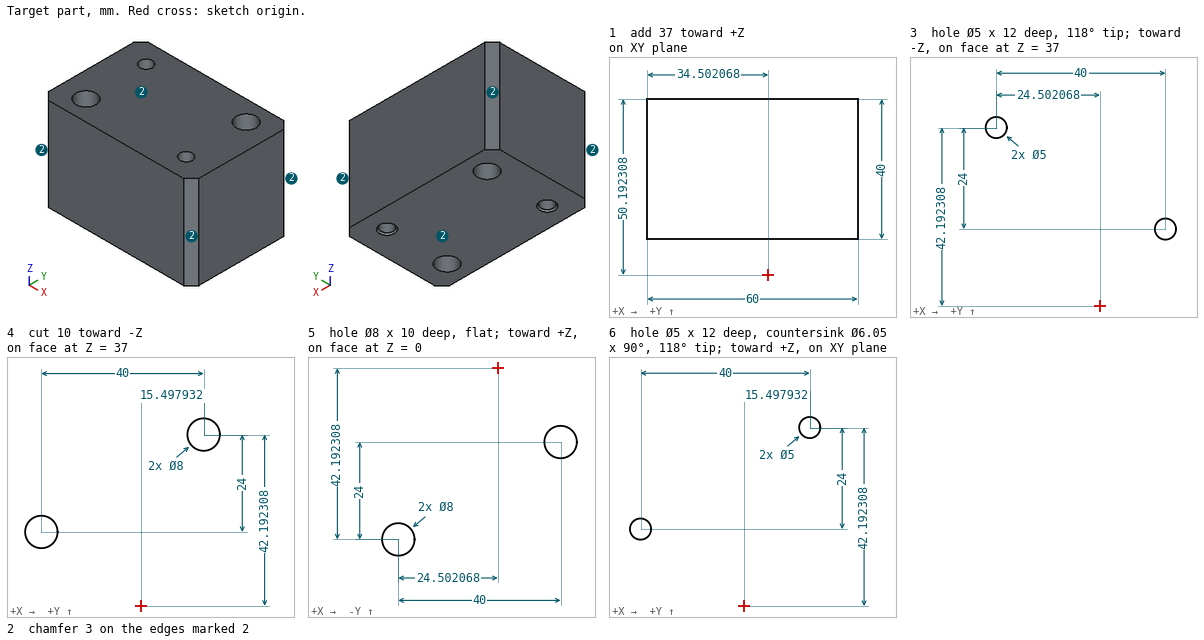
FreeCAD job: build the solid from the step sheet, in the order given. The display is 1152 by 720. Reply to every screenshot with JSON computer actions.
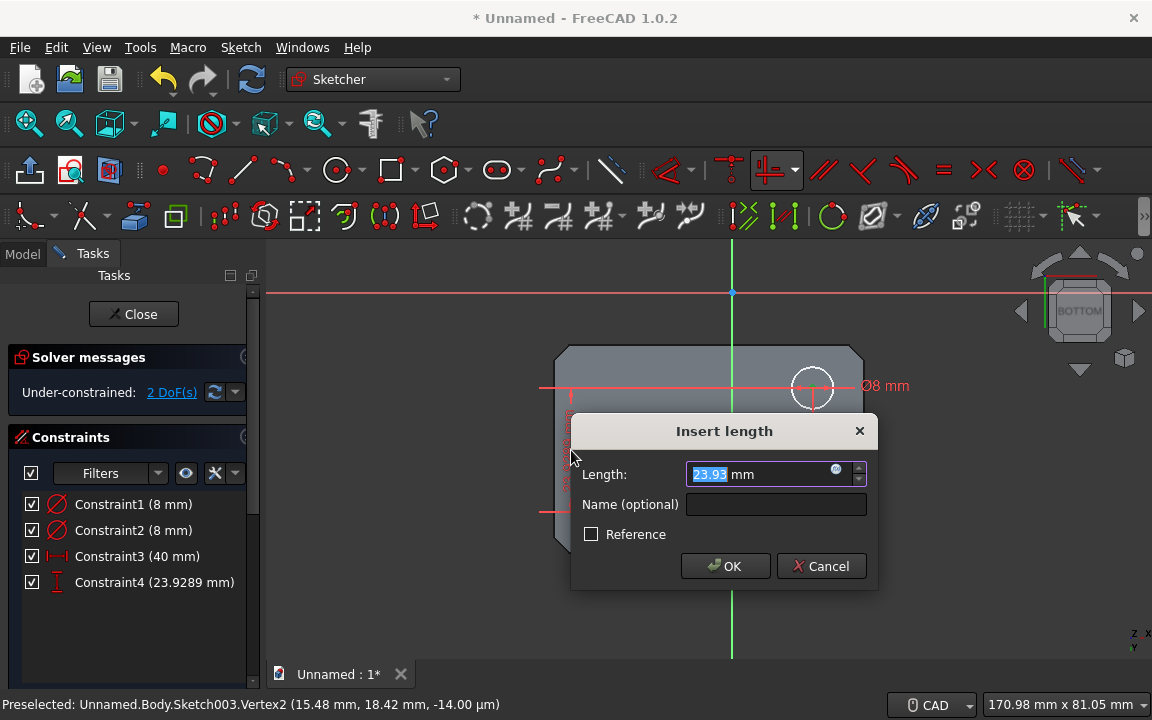
{"action": "type", "text": "24"}
{"action": "key", "text": "Return"}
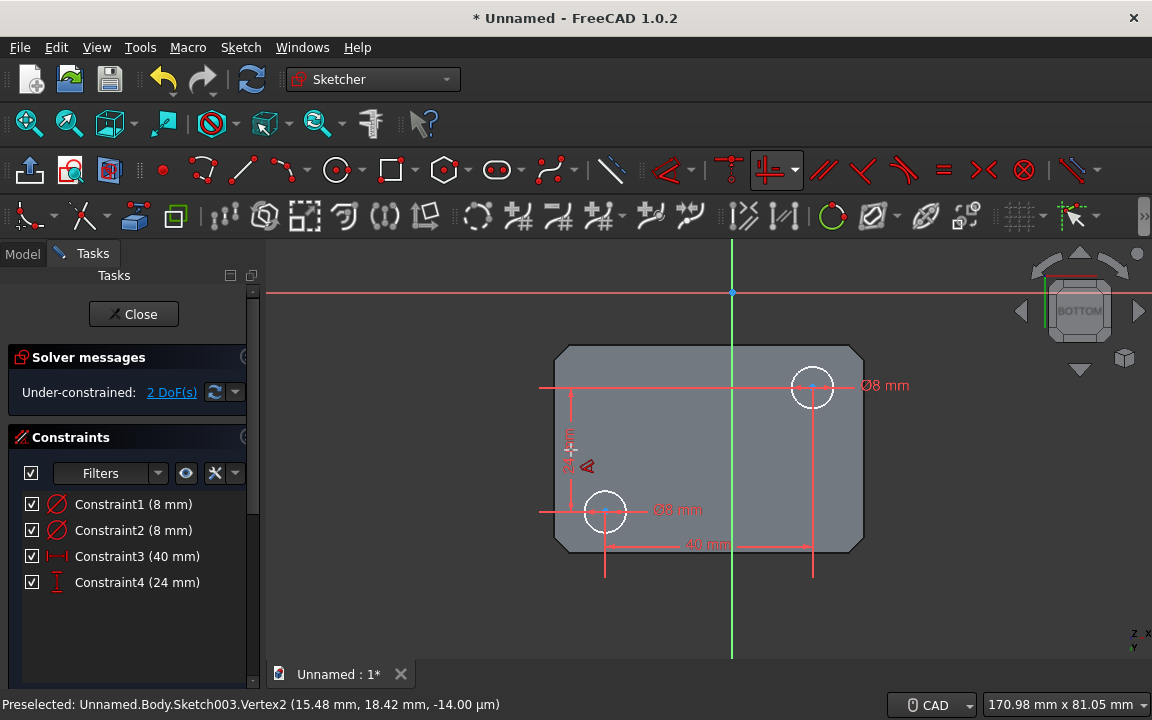
{"action": "left_click", "coordinate": [605, 512]}
{"action": "left_click", "coordinate": [624, 546]}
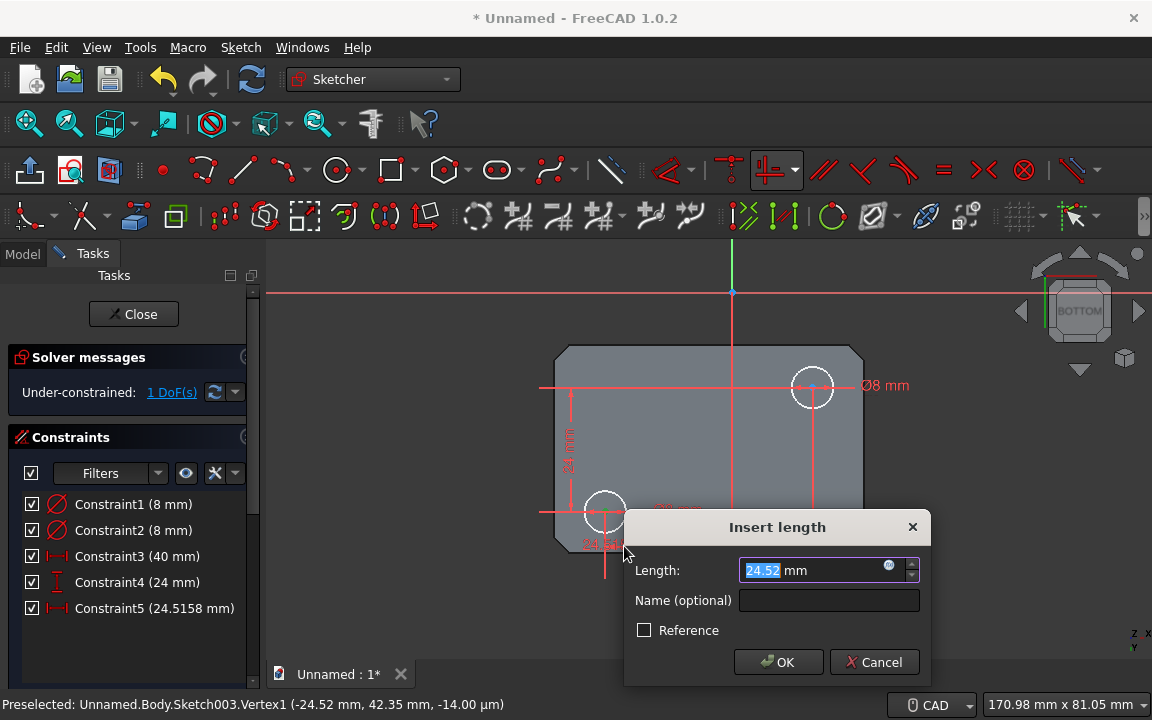
{"action": "type", "text": "24.502068"}
{"action": "key", "text": "Return"}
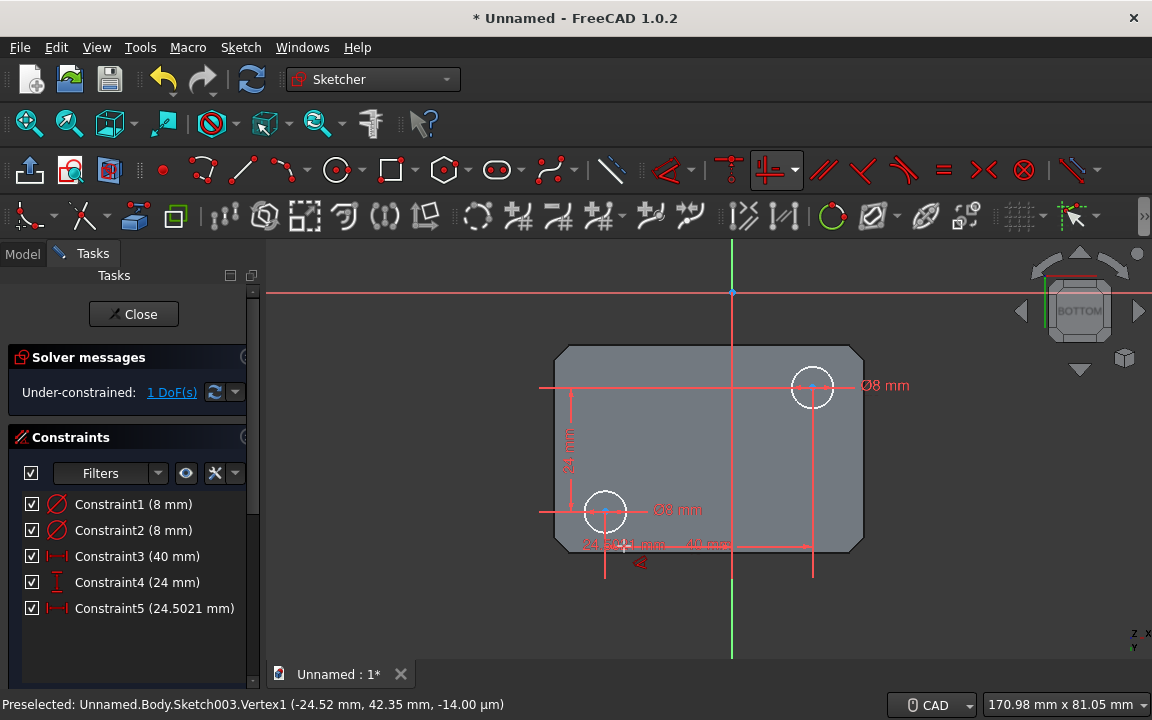
{"action": "left_click", "coordinate": [605, 512]}
{"action": "left_click", "coordinate": [571, 402]}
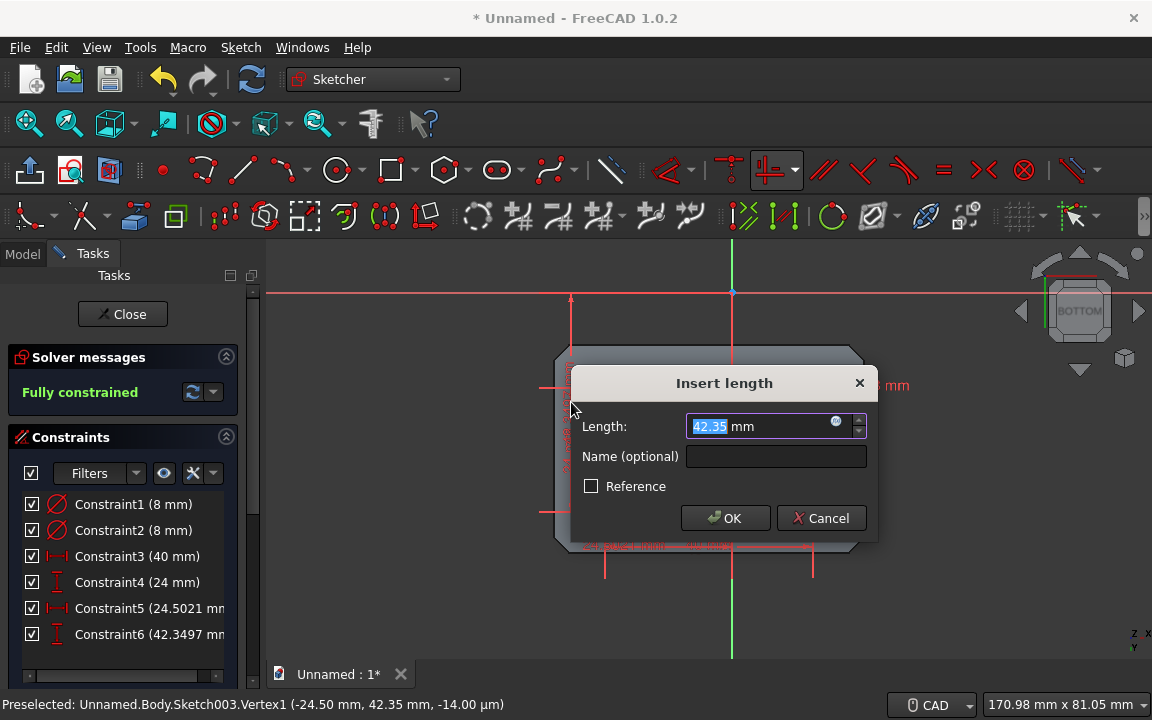
{"action": "type", "text": "42.192308"}
{"action": "key", "text": "Return"}
{"action": "key", "text": "Escape"}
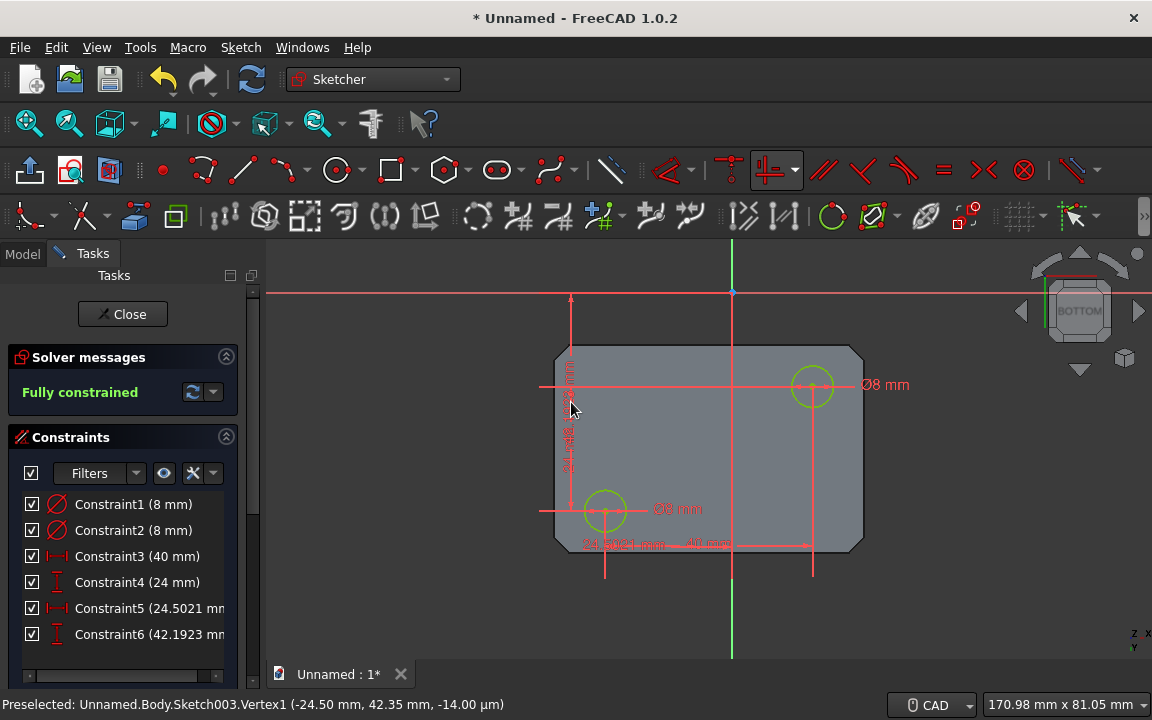
{"action": "left_click", "coordinate": [123, 314]}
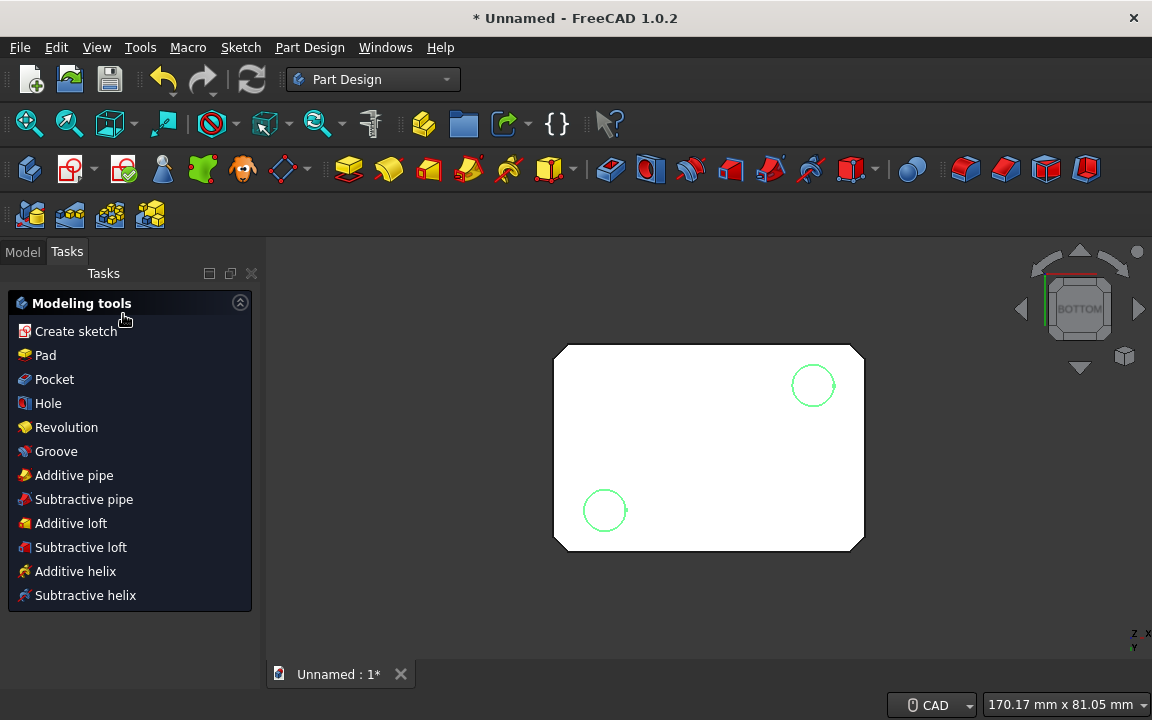
{"action": "left_click", "coordinate": [652, 170]}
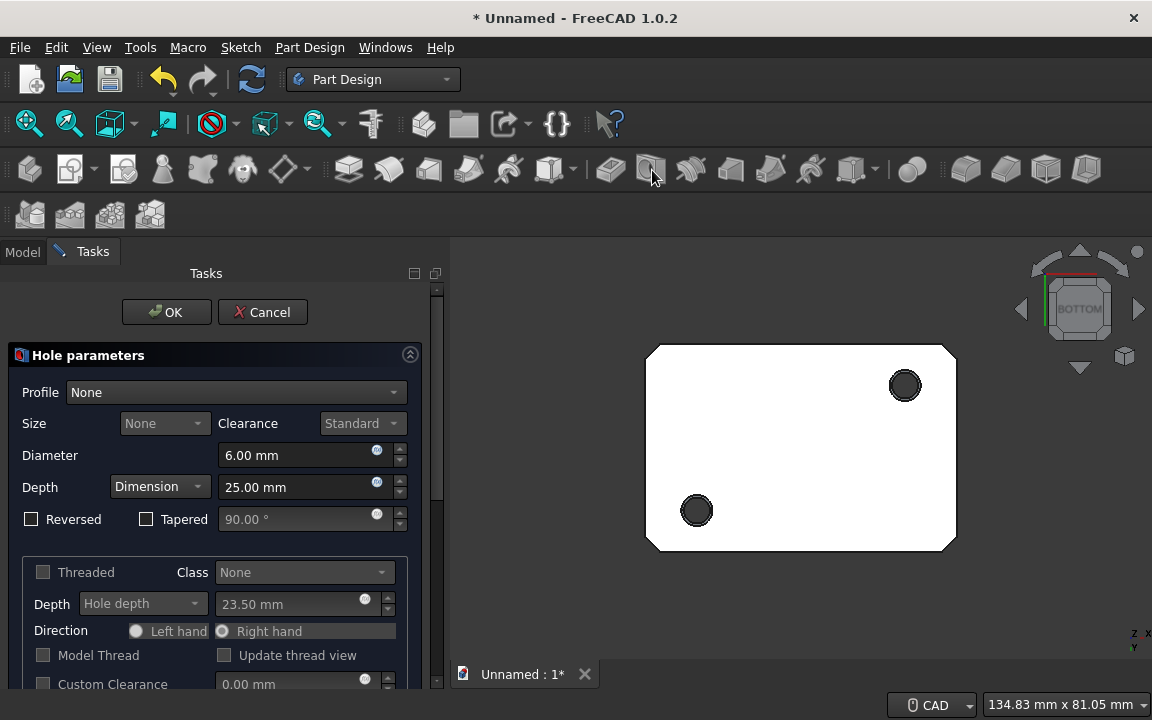
{"action": "triple_click", "coordinate": [305, 455]}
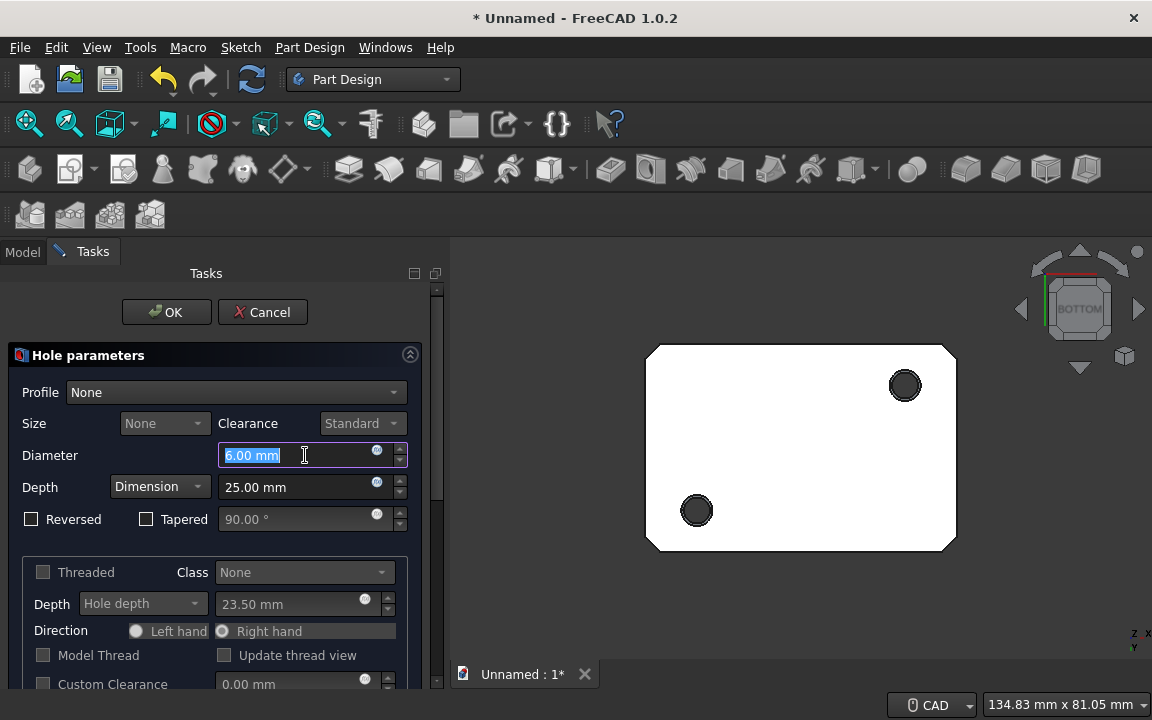
{"action": "type", "text": "8"}
{"action": "key", "text": "Tab"}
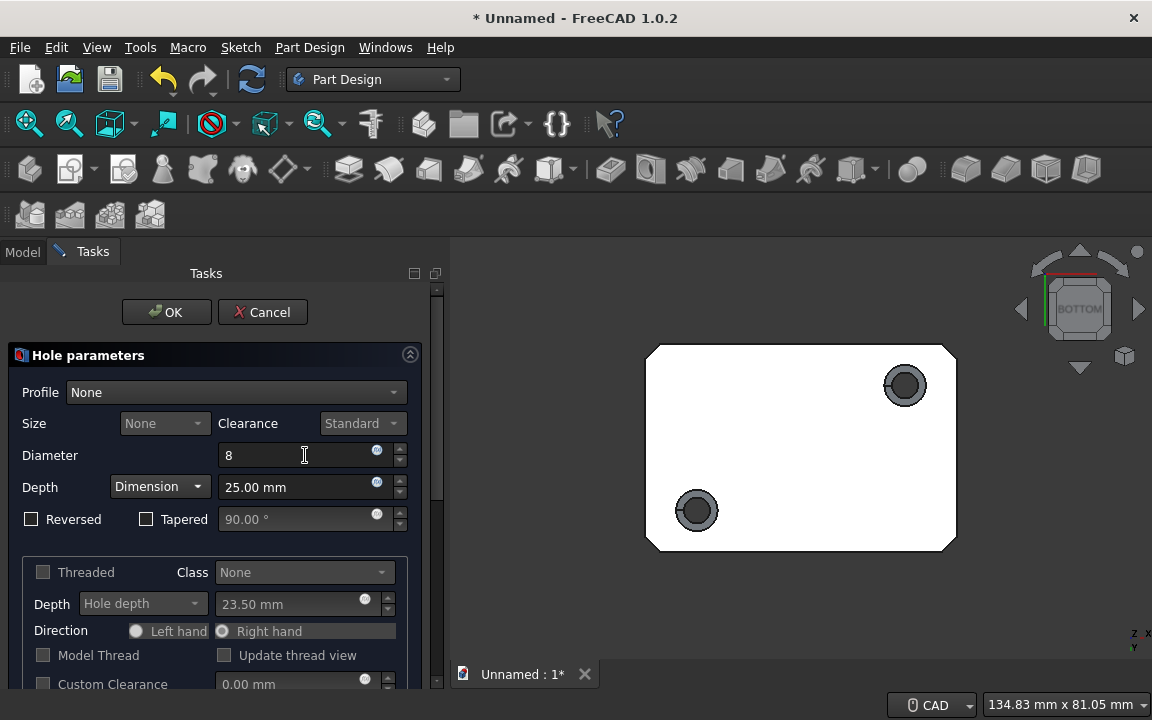
{"action": "triple_click", "coordinate": [305, 487]}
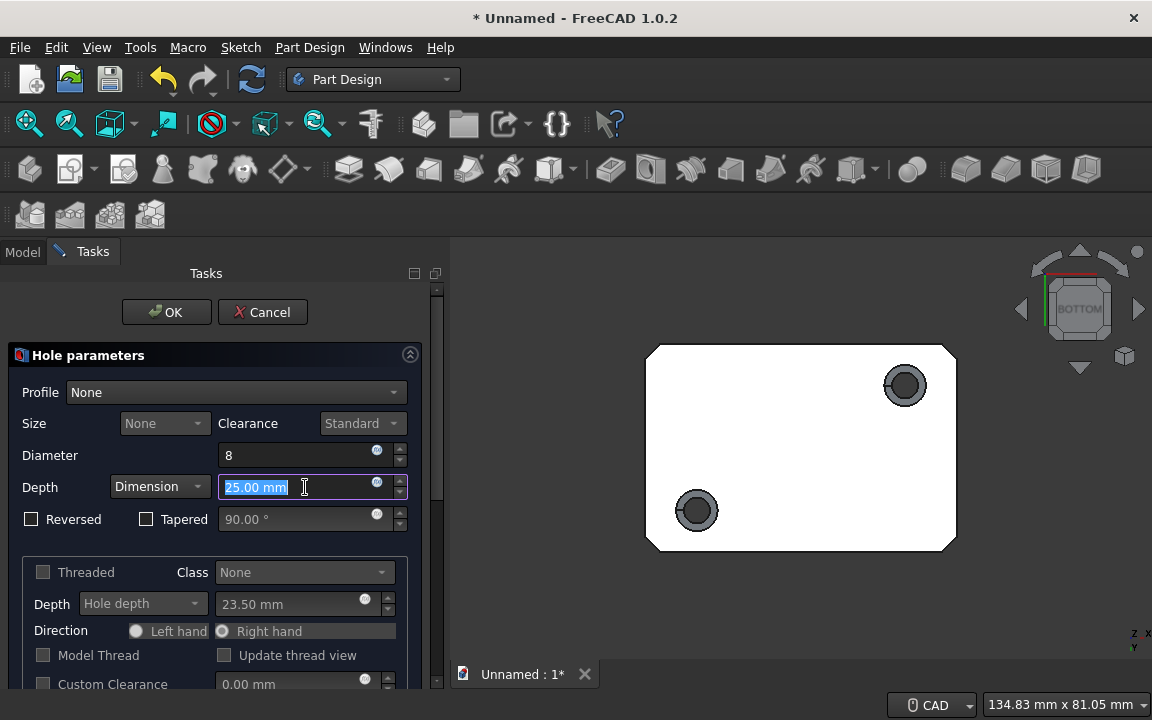
{"action": "type", "text": "10"}
{"action": "key", "text": "Tab"}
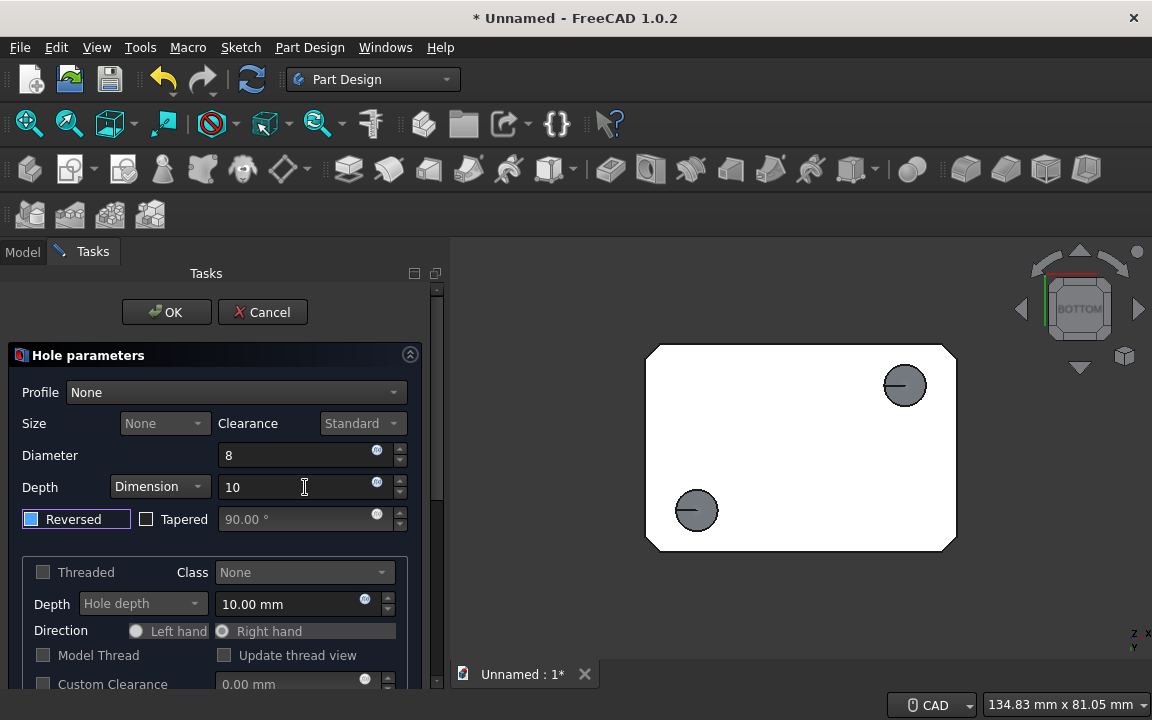
{"action": "scroll", "coordinate": [437, 486], "scroll_direction": "down", "scroll_amount": 6}